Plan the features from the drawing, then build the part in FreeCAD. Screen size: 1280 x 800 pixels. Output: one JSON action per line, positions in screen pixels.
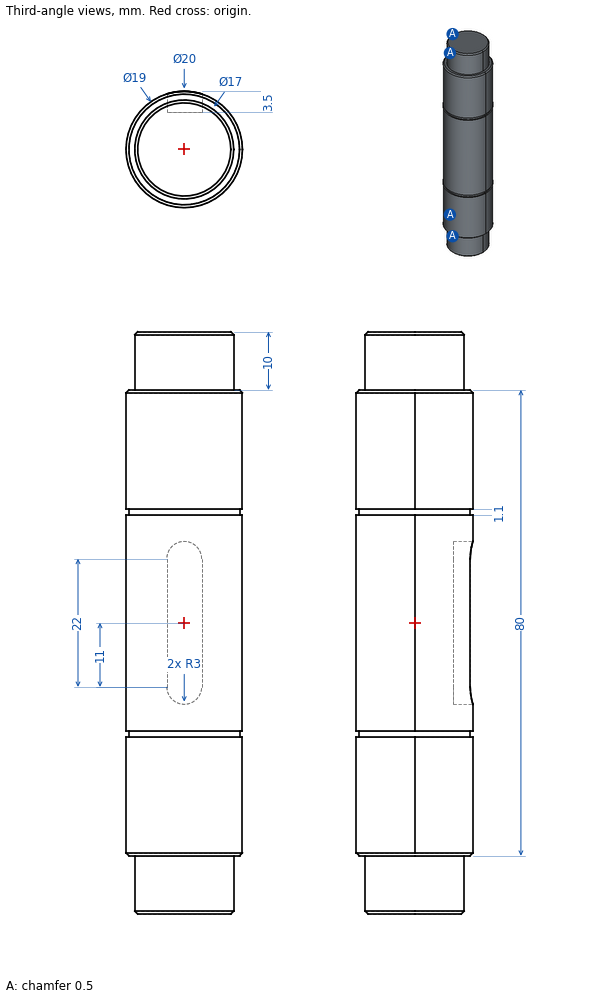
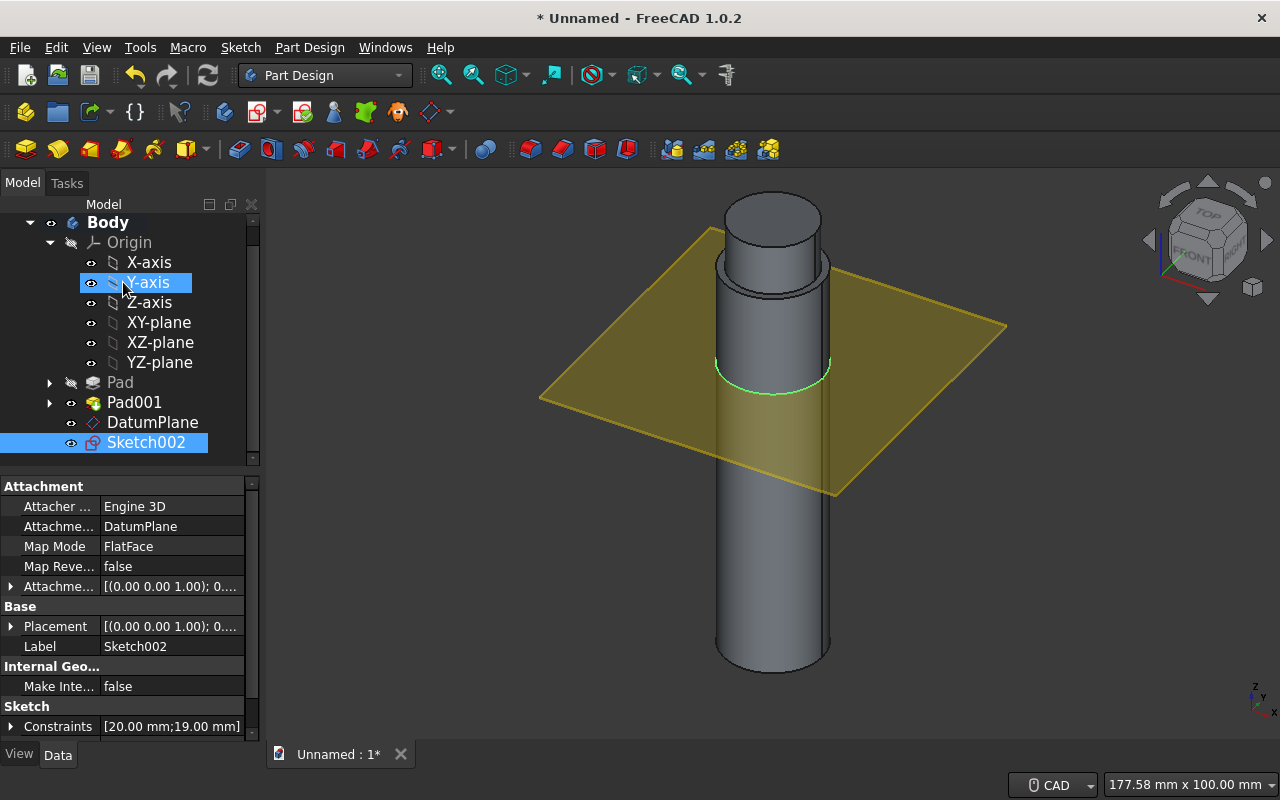
{"action": "left_click", "coordinate": [240, 150]}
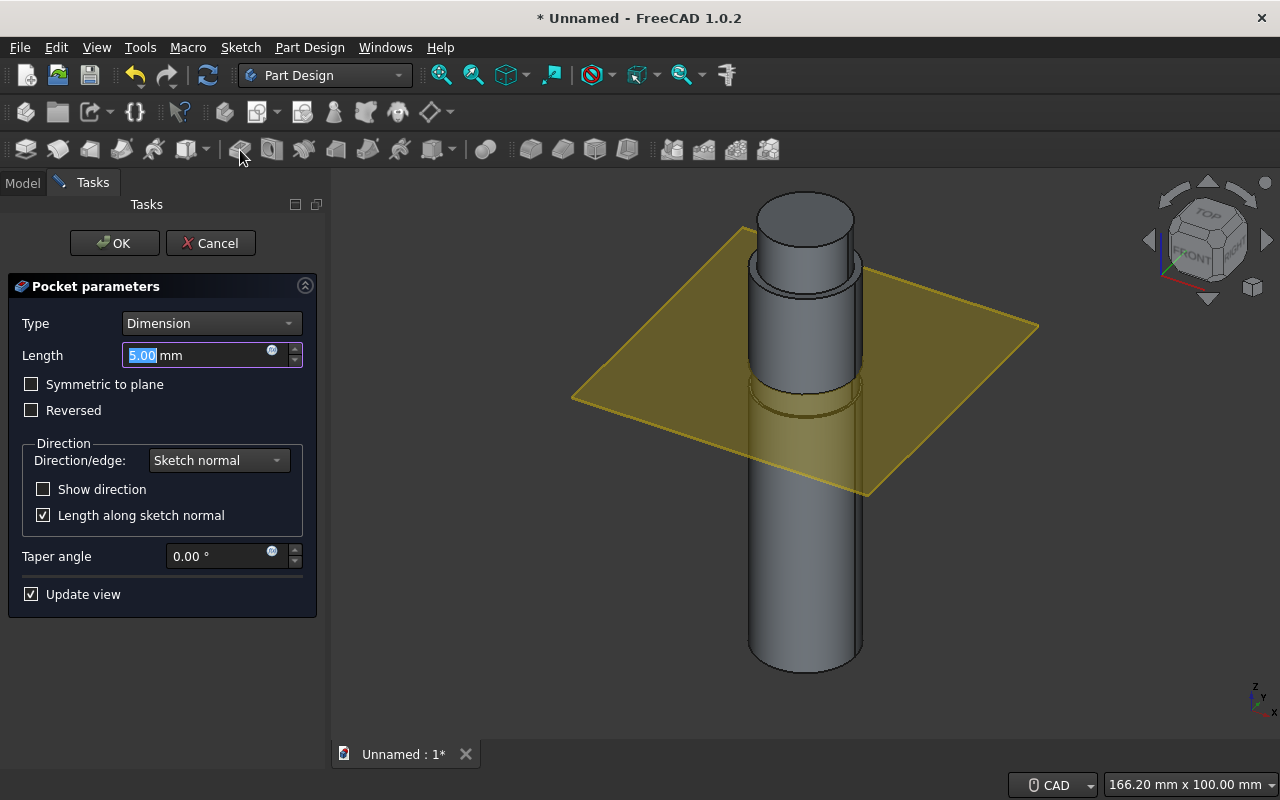
{"action": "type", "text": "1.1"}
{"action": "key", "text": "Tab"}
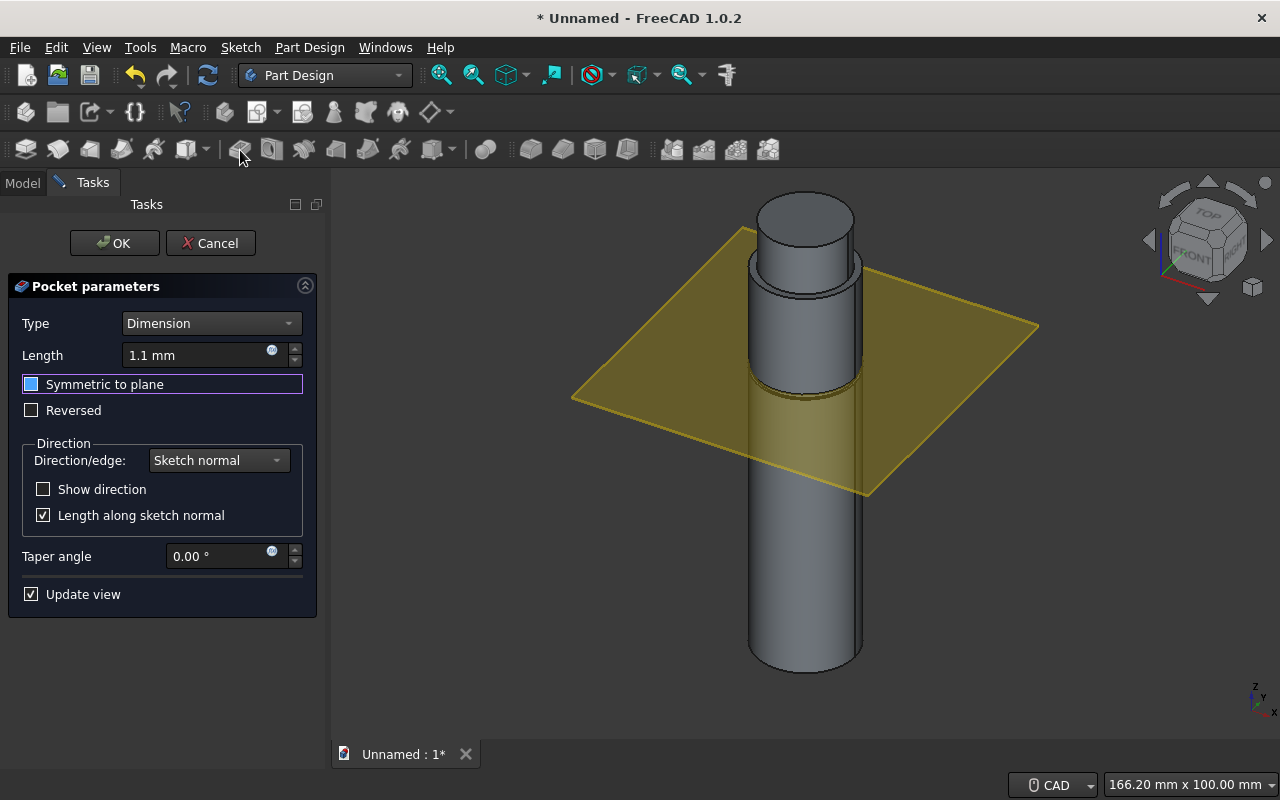
{"action": "left_click", "coordinate": [115, 243]}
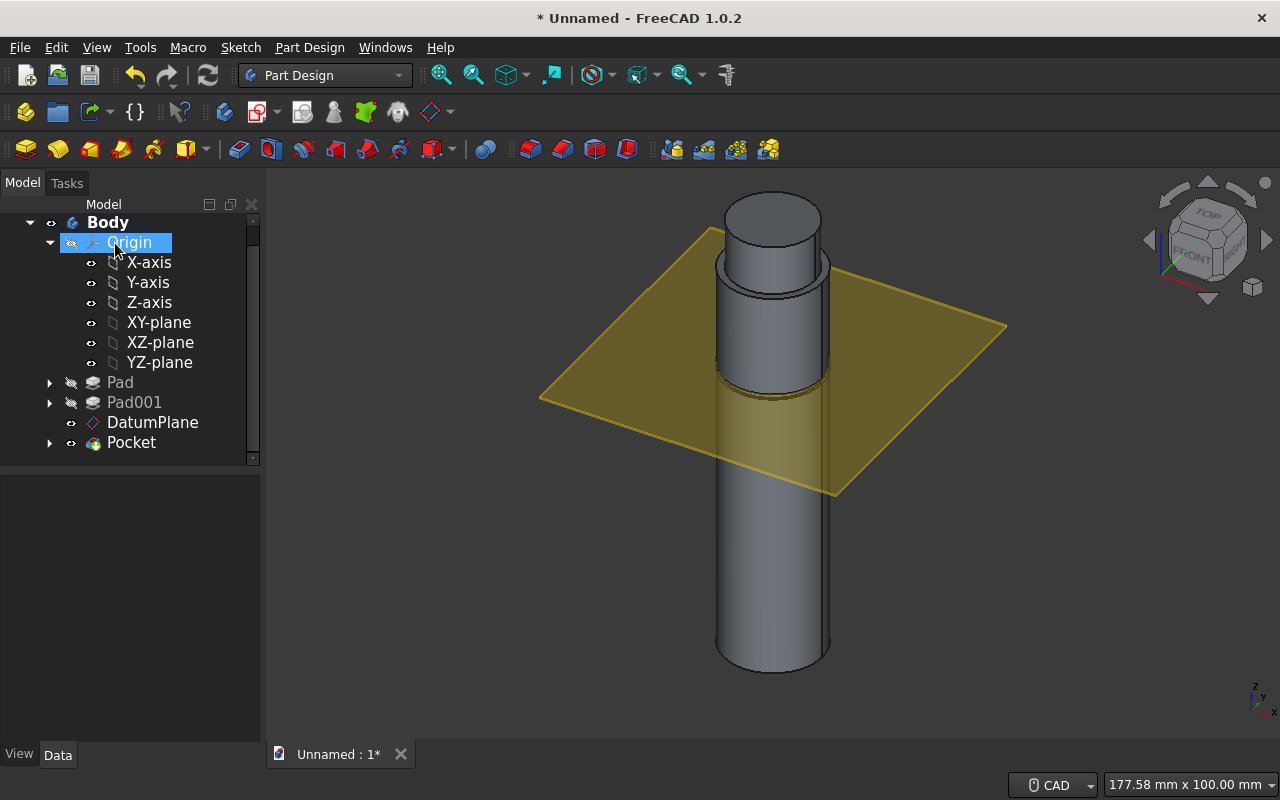
{"action": "left_click", "coordinate": [116, 423]}
{"action": "key", "text": "space"}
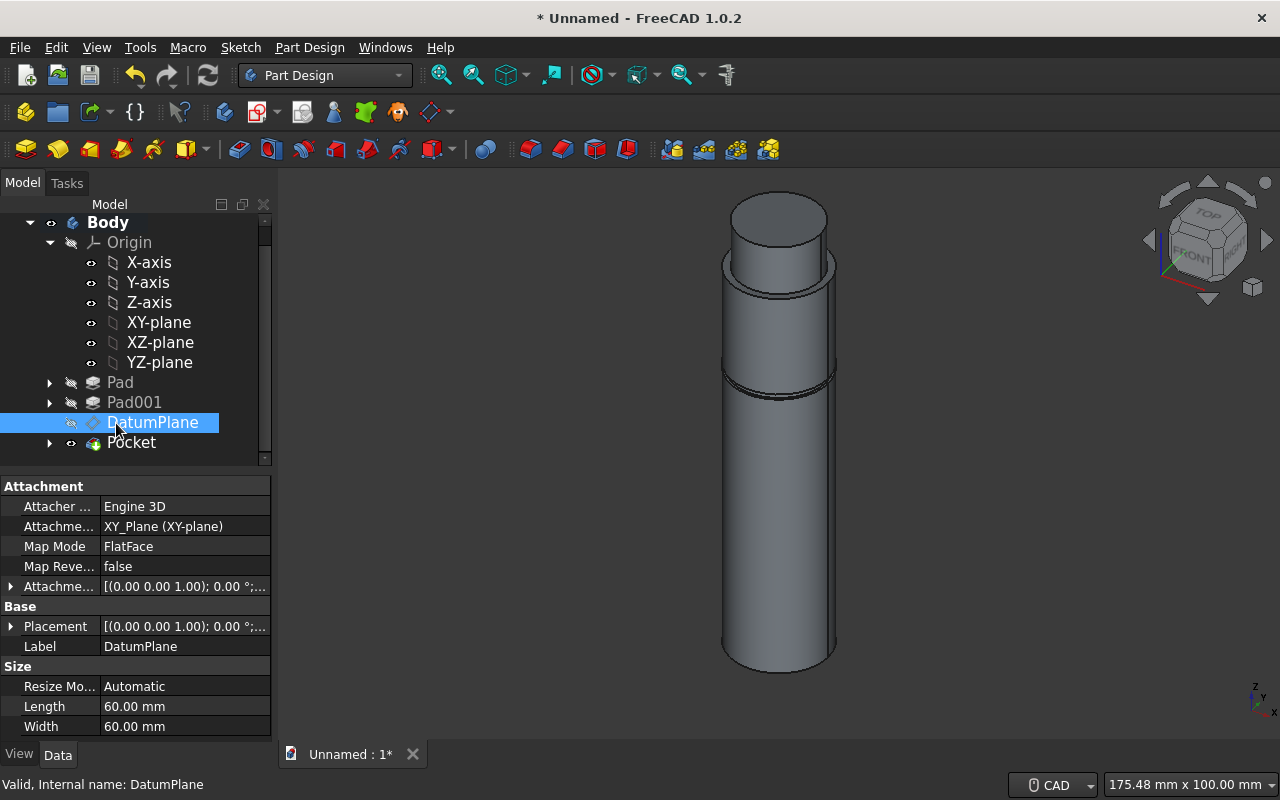
{"action": "left_click", "coordinate": [116, 403]}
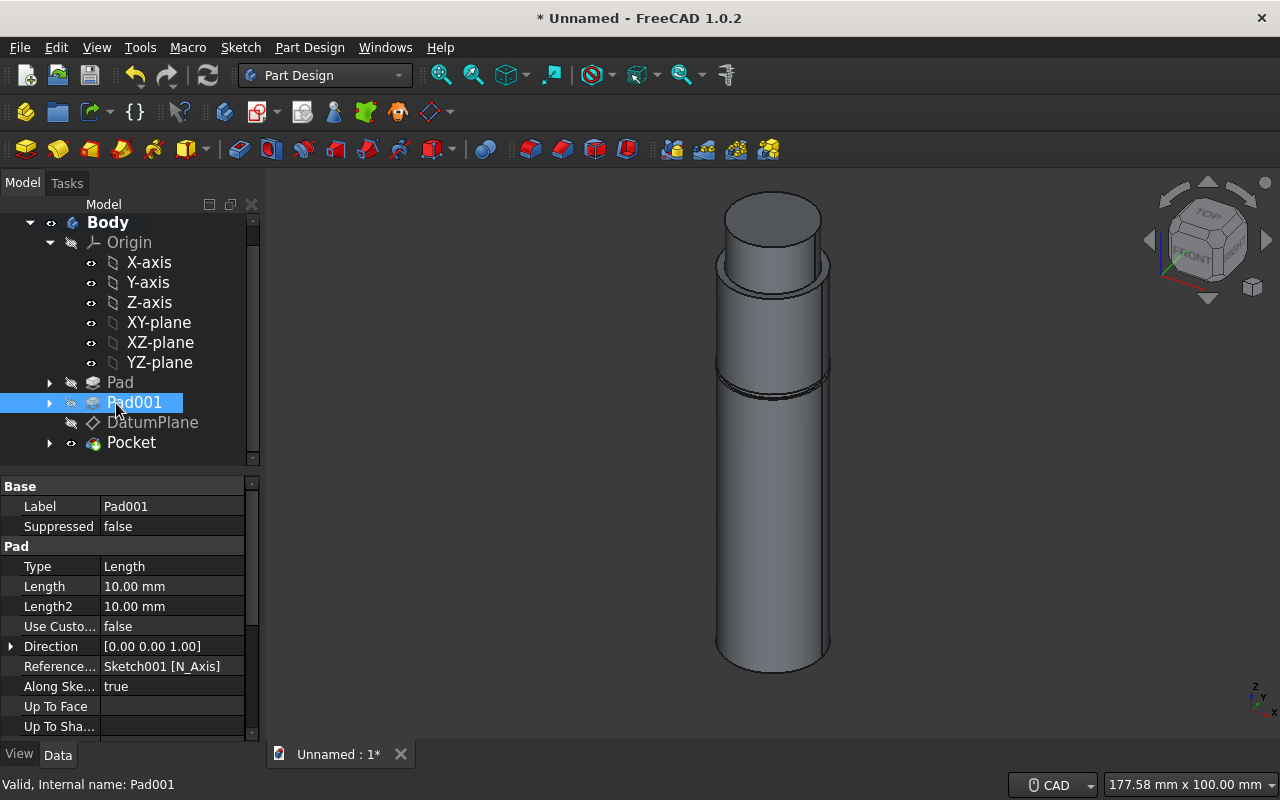
{"action": "left_click", "coordinate": [116, 443], "text": "ctrl"}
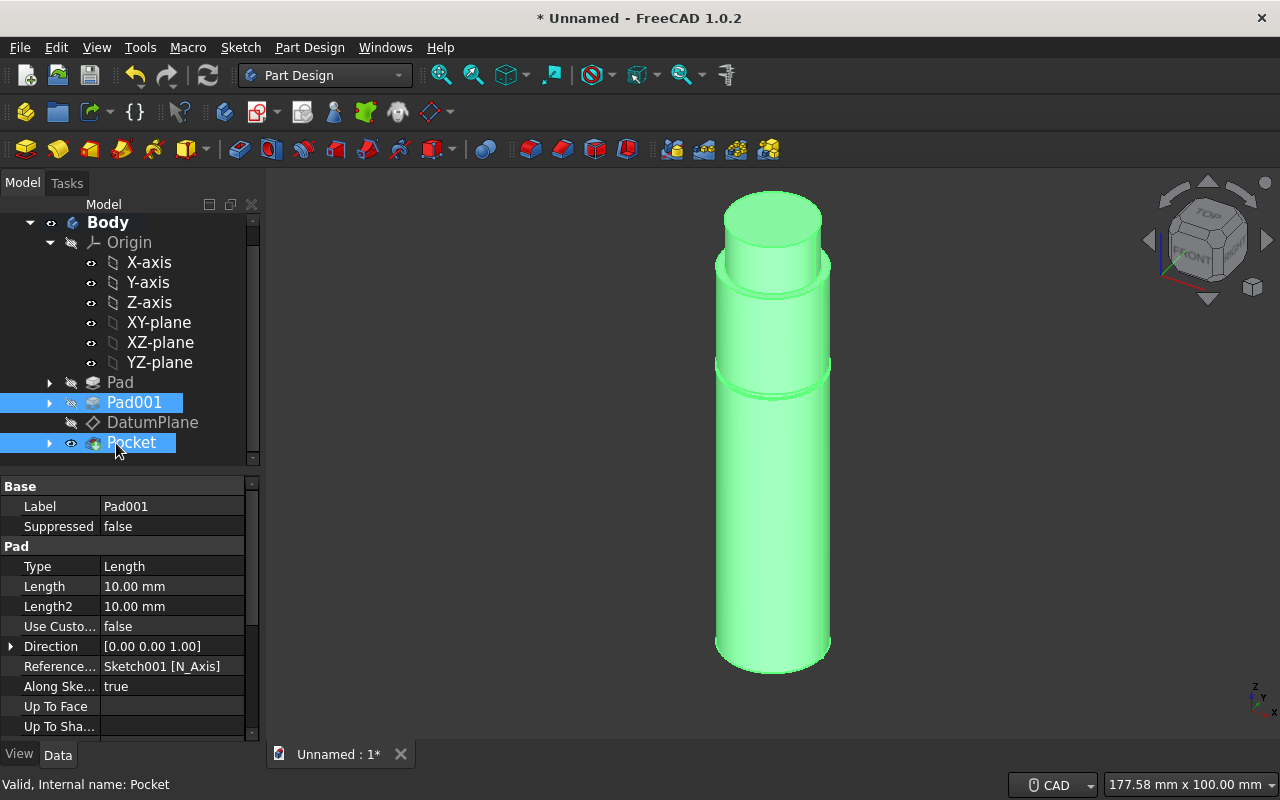
{"action": "left_click", "coordinate": [672, 150]}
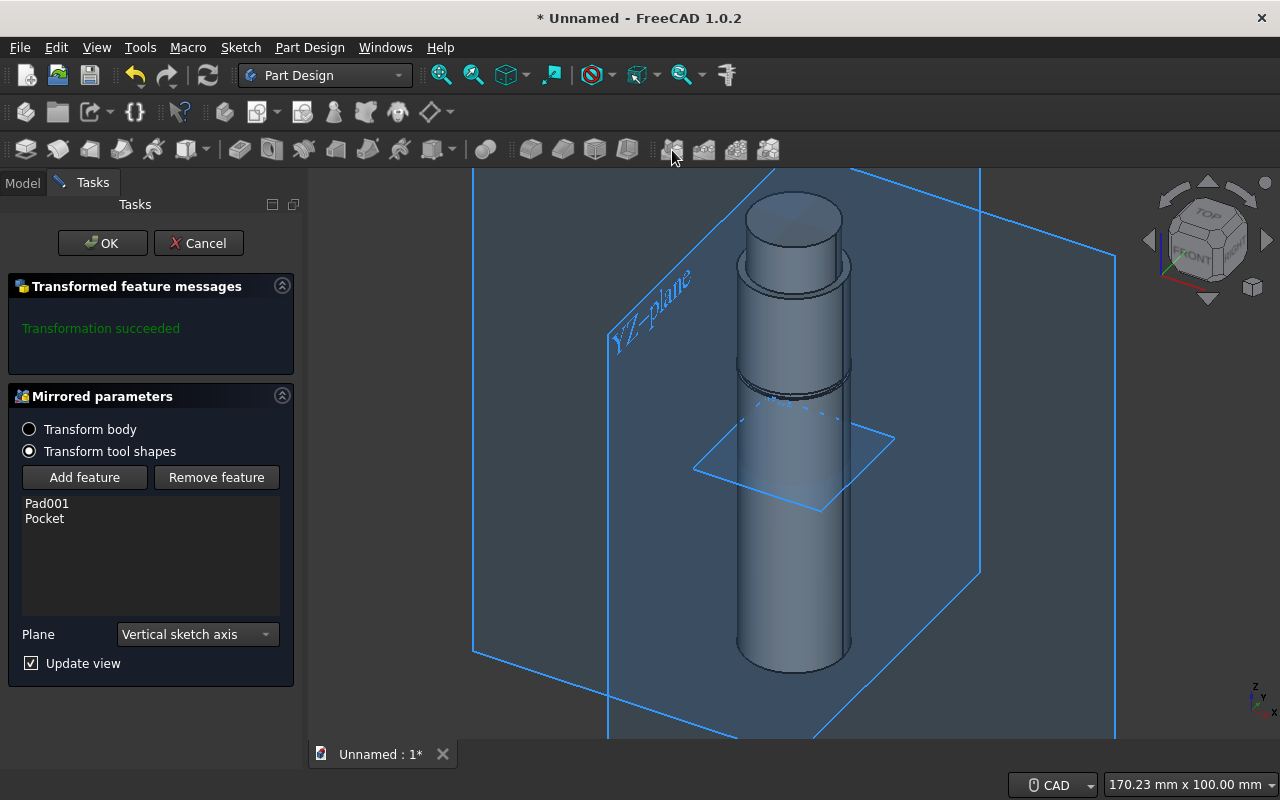
{"action": "left_click", "coordinate": [198, 634]}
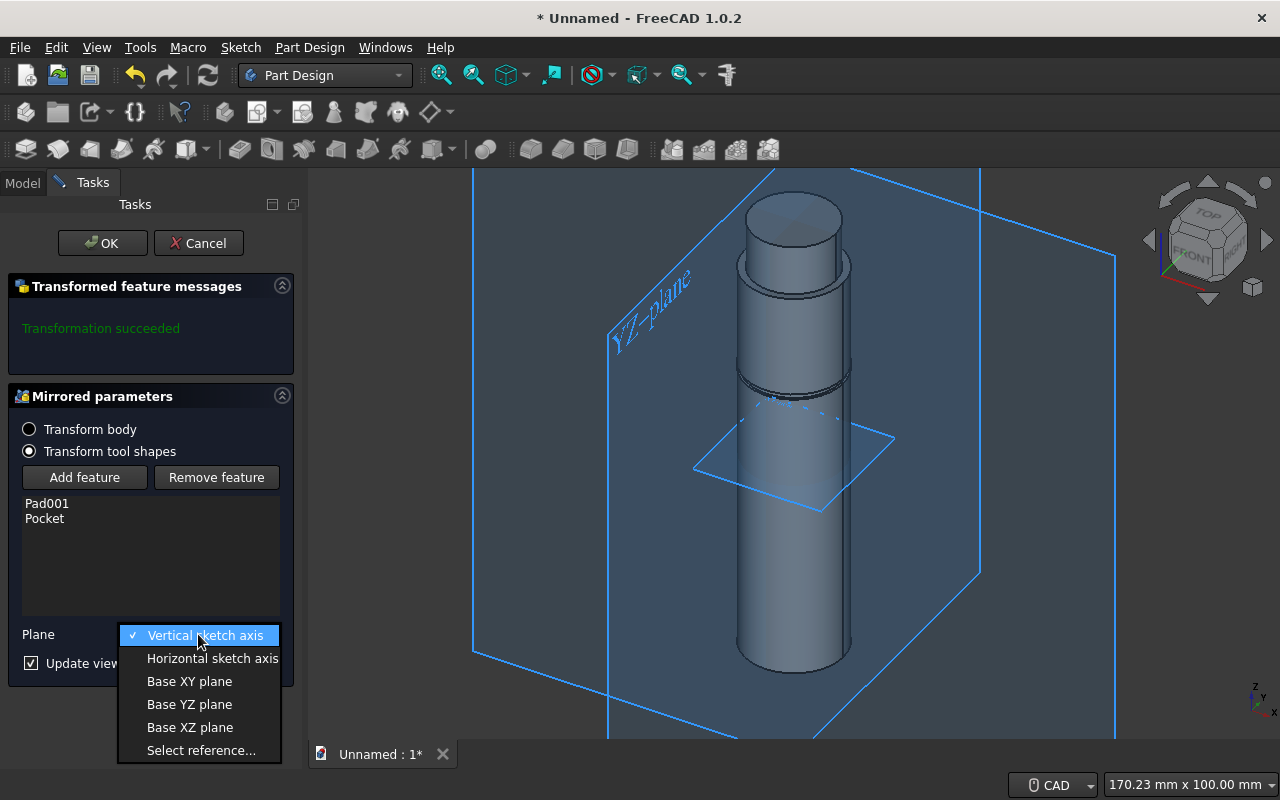
{"action": "left_click", "coordinate": [198, 682]}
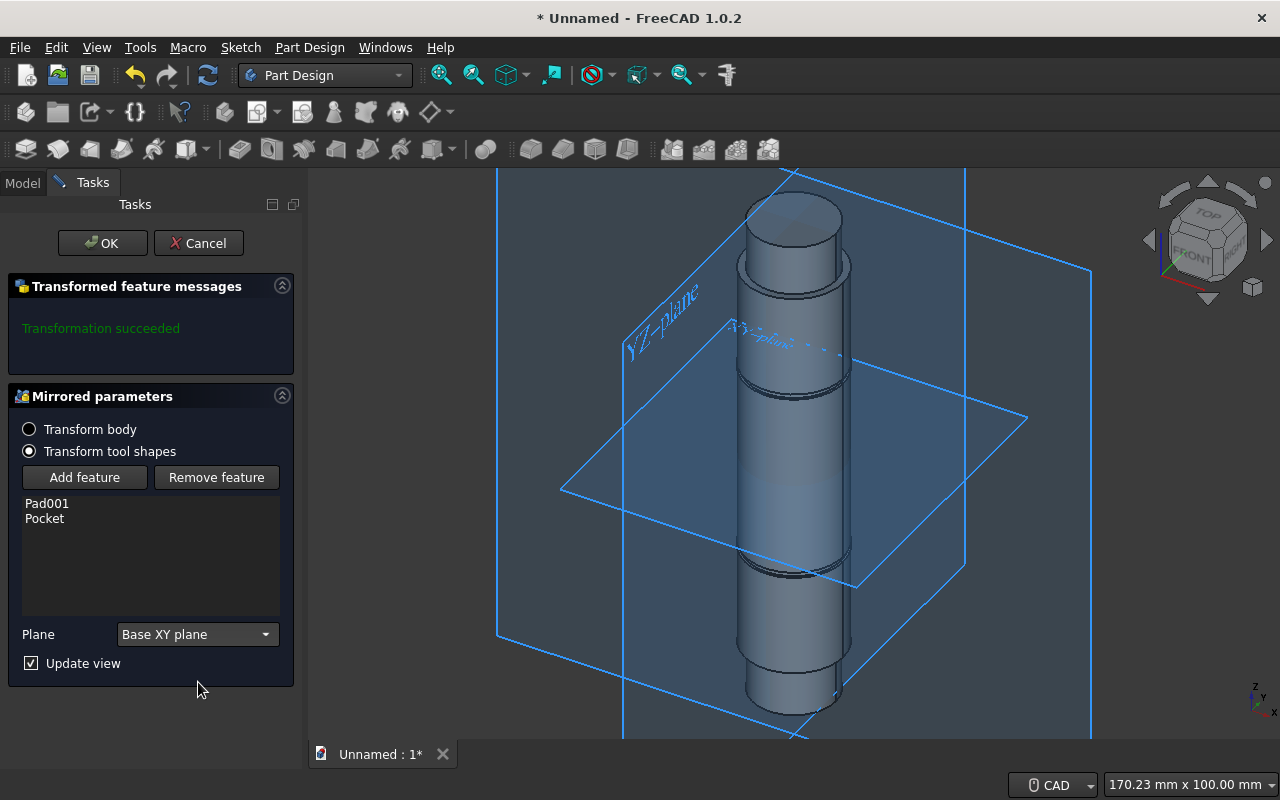
{"action": "left_click", "coordinate": [103, 243]}